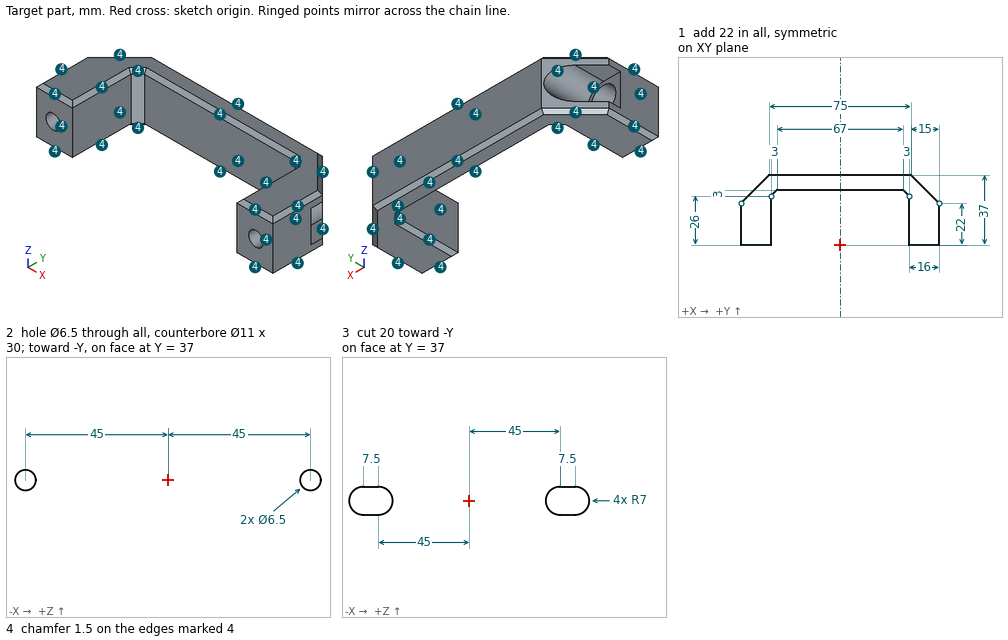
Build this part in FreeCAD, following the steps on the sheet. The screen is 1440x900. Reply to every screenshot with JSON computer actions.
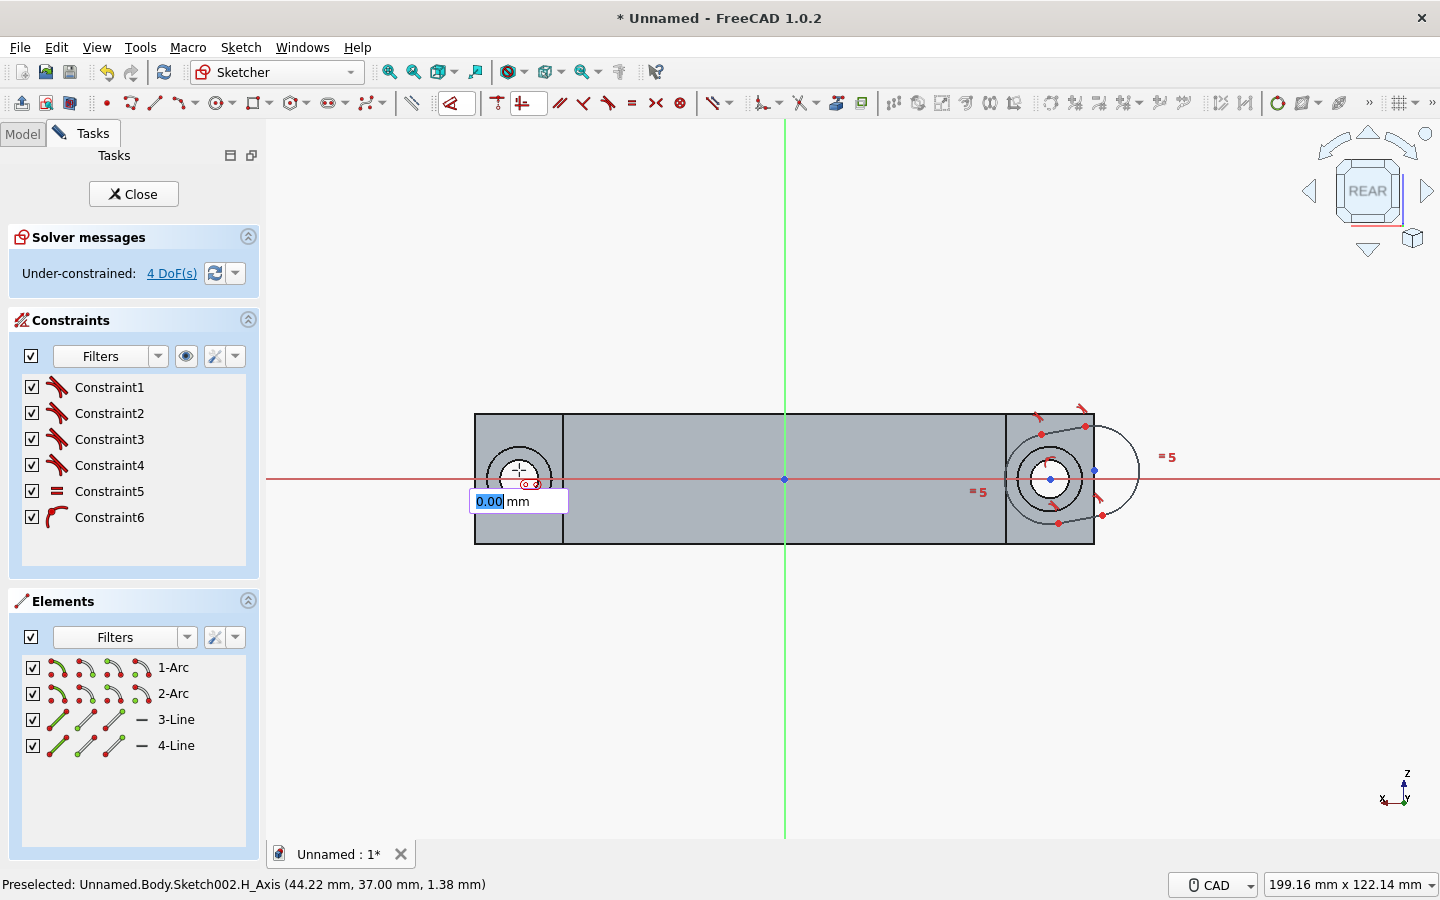
{"action": "left_click", "coordinate": [497, 520]}
{"action": "key", "text": "Escape"}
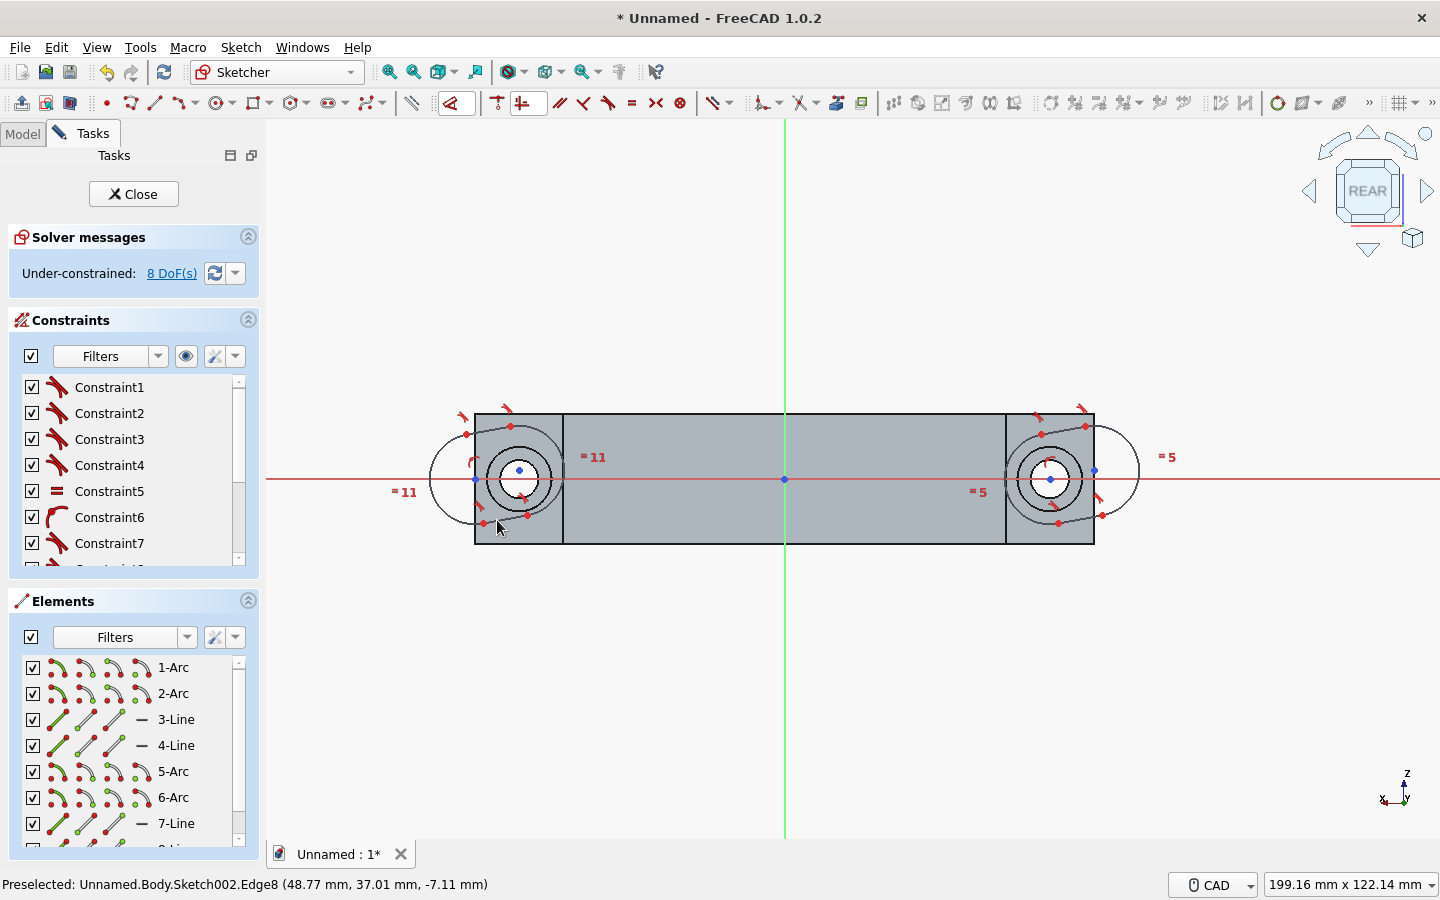
{"action": "left_click", "coordinate": [1055, 432]}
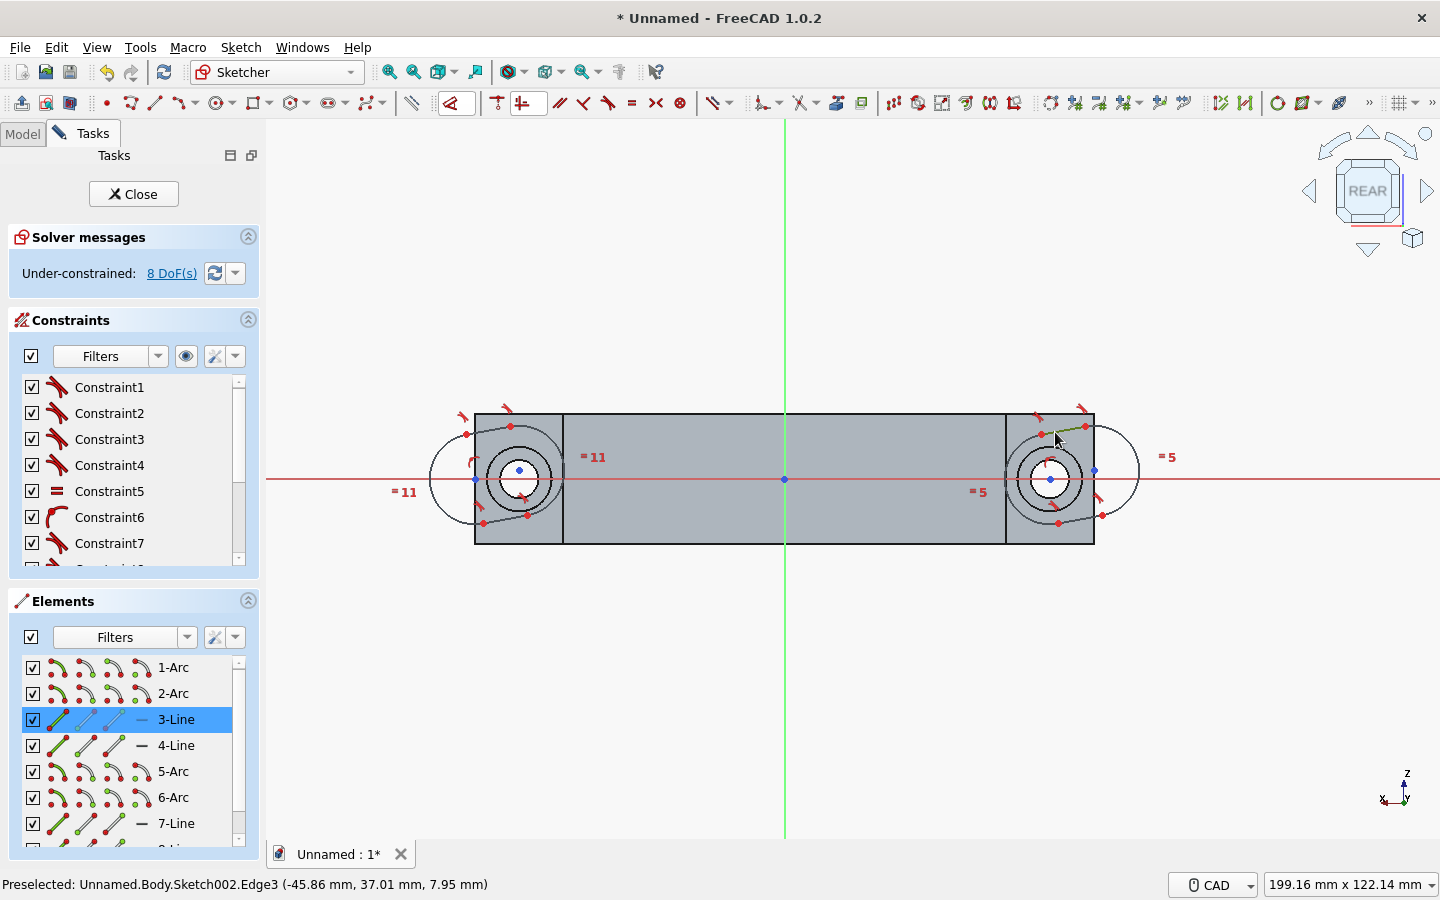
{"action": "key", "text": "h"}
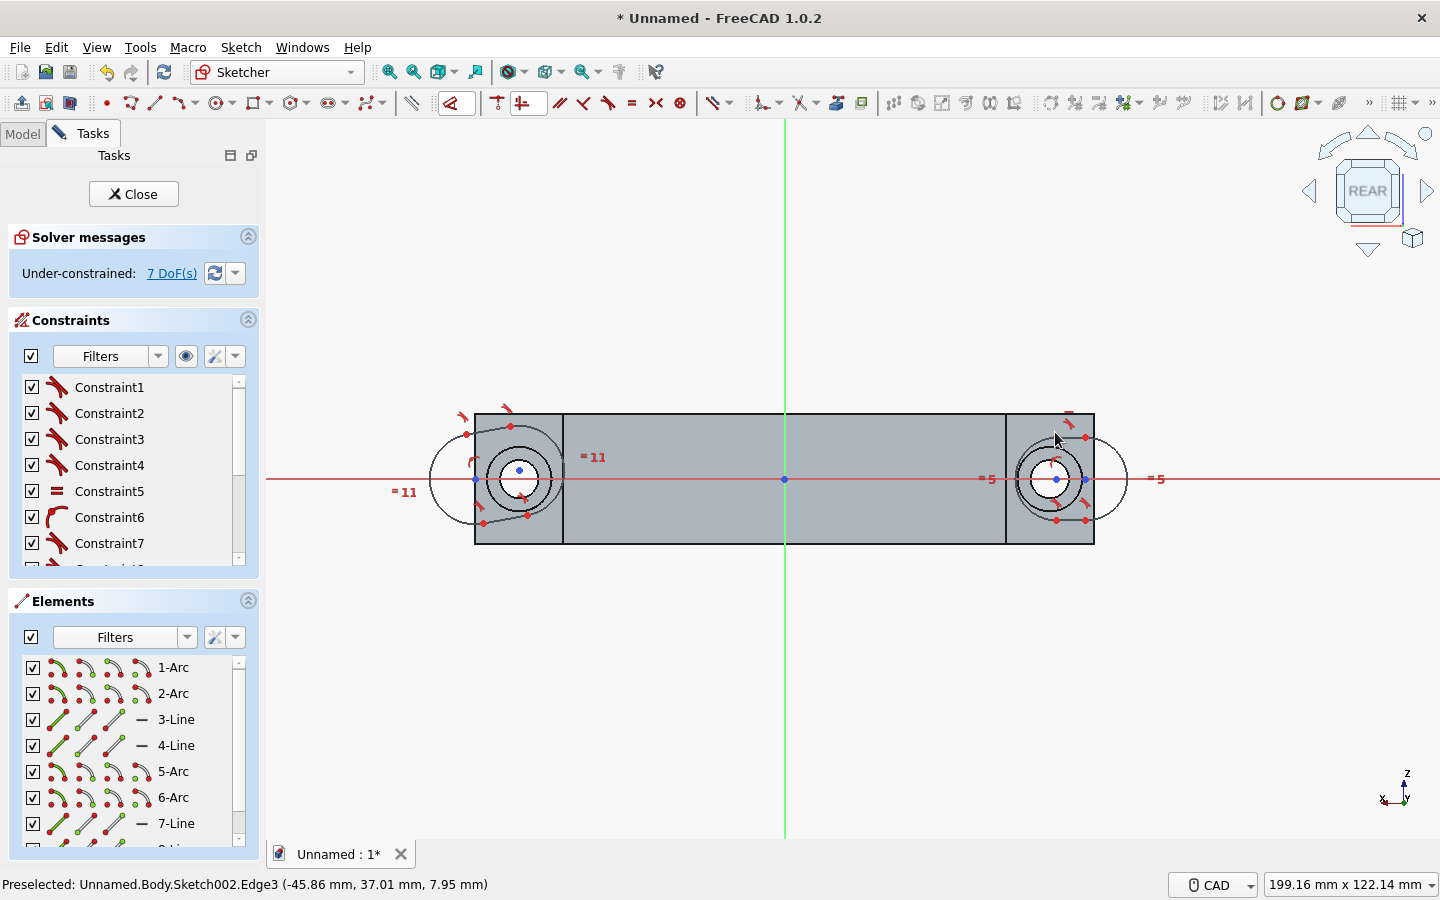
{"action": "left_click", "coordinate": [480, 432]}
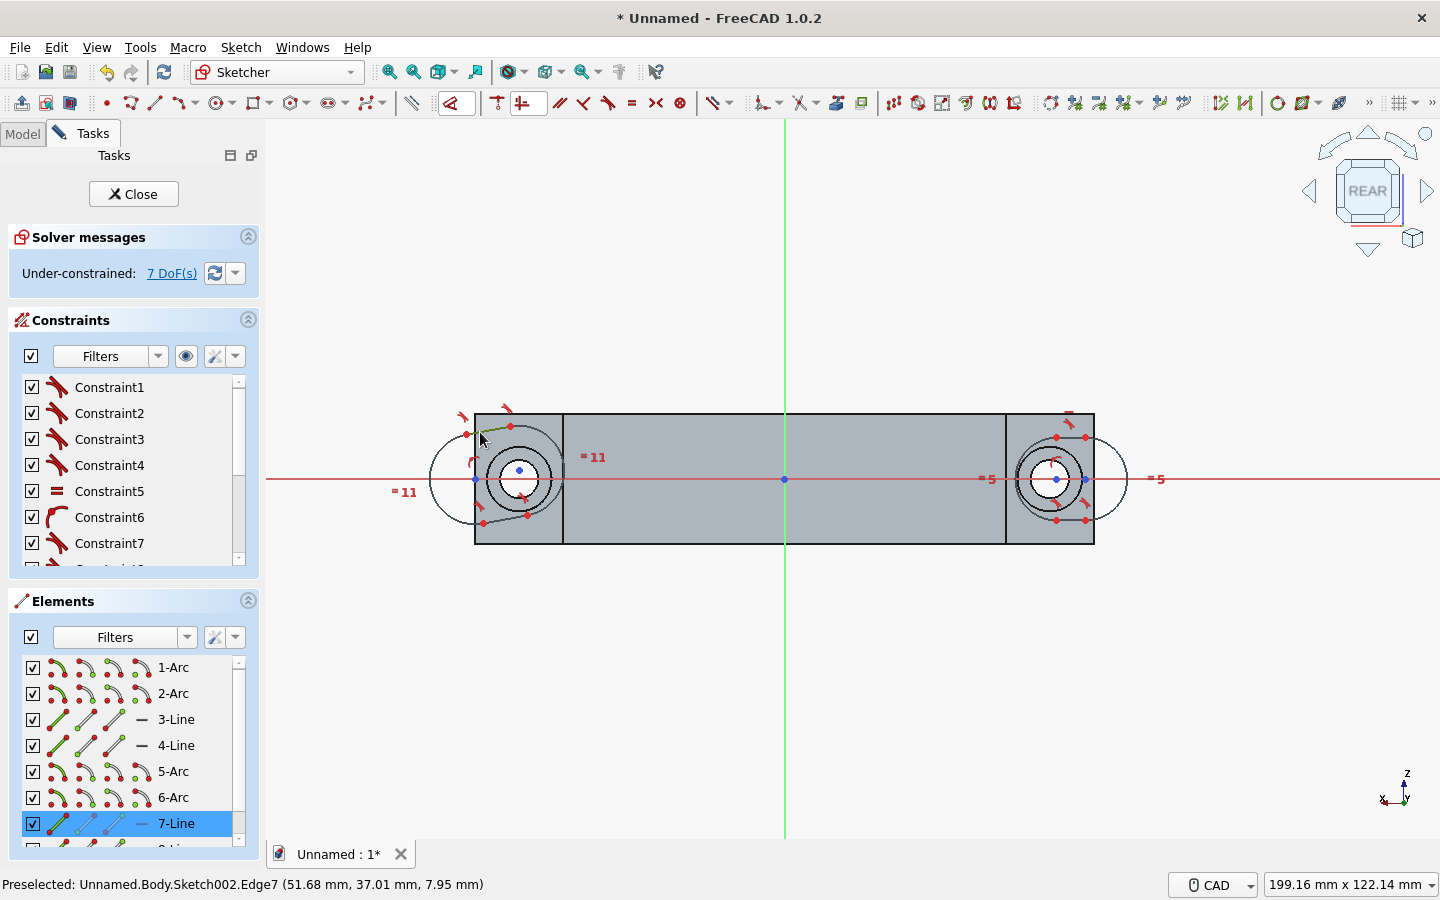
{"action": "left_click", "coordinate": [542, 104]}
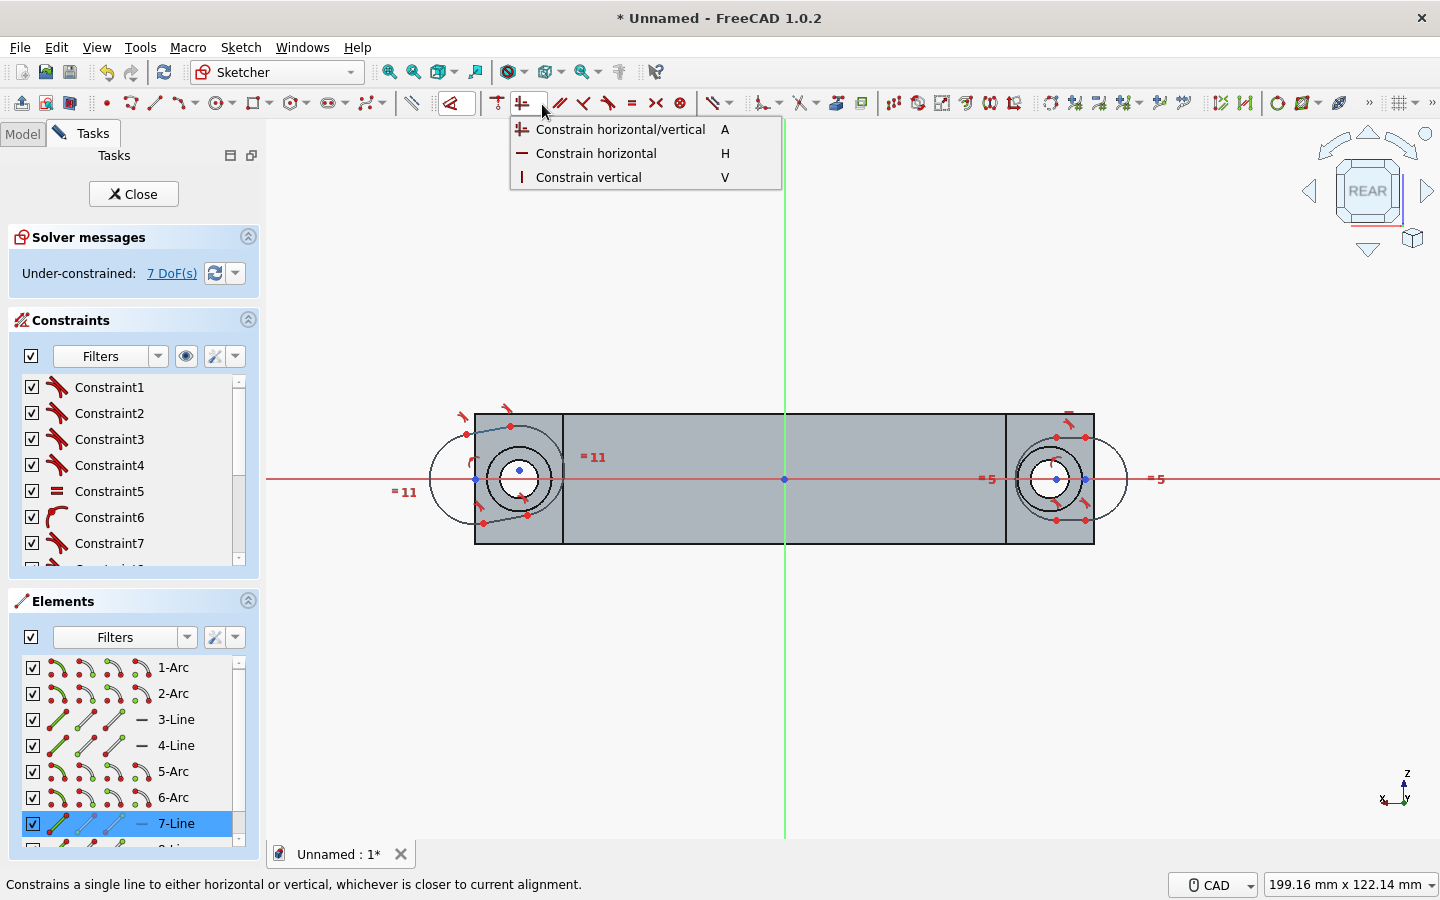
{"action": "left_click", "coordinate": [646, 153]}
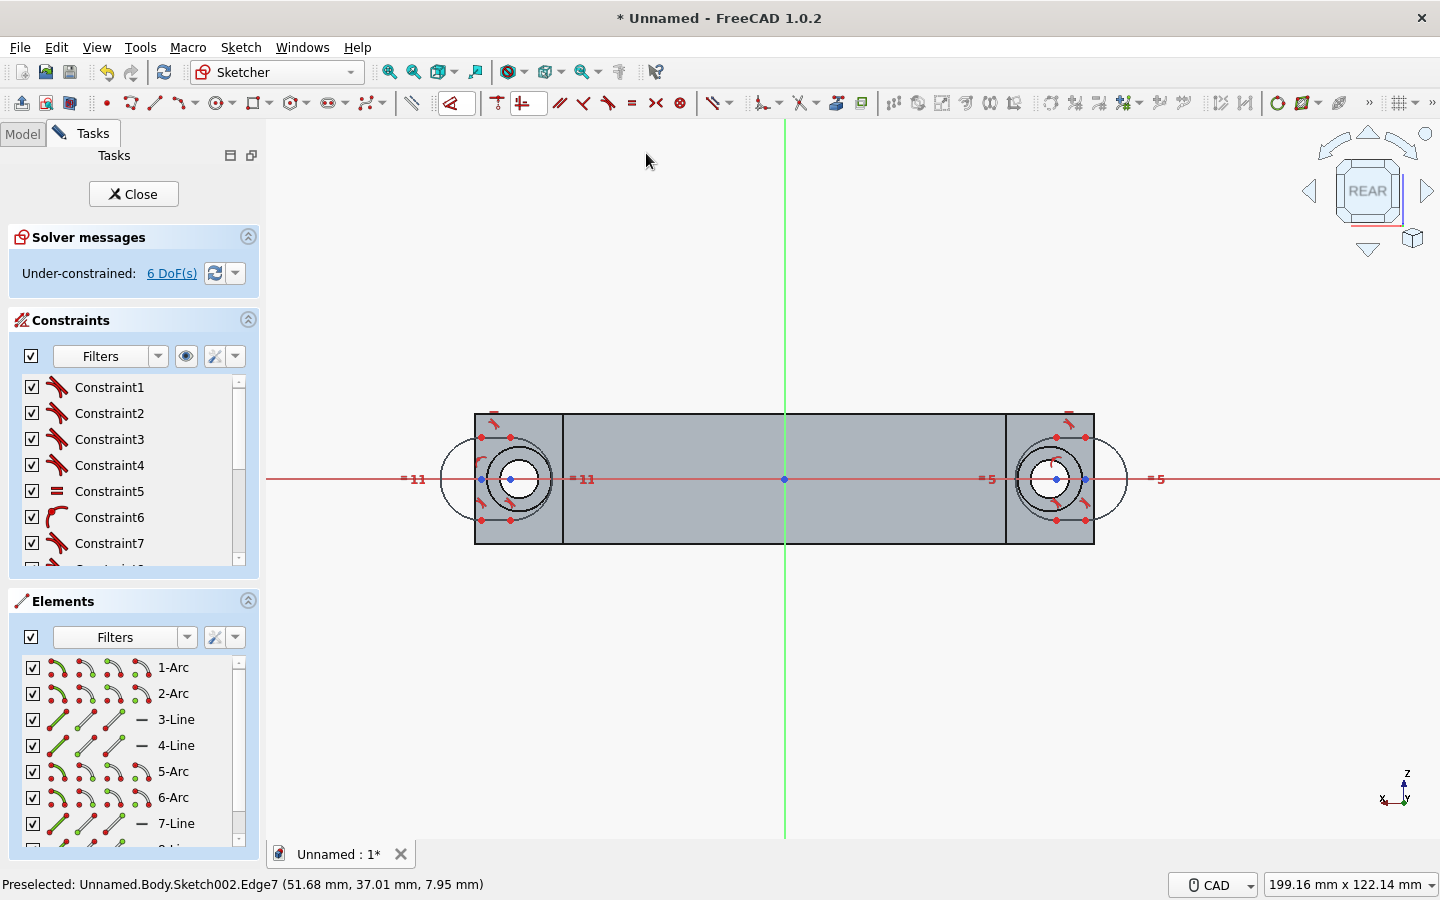
{"action": "left_click", "coordinate": [1023, 455]}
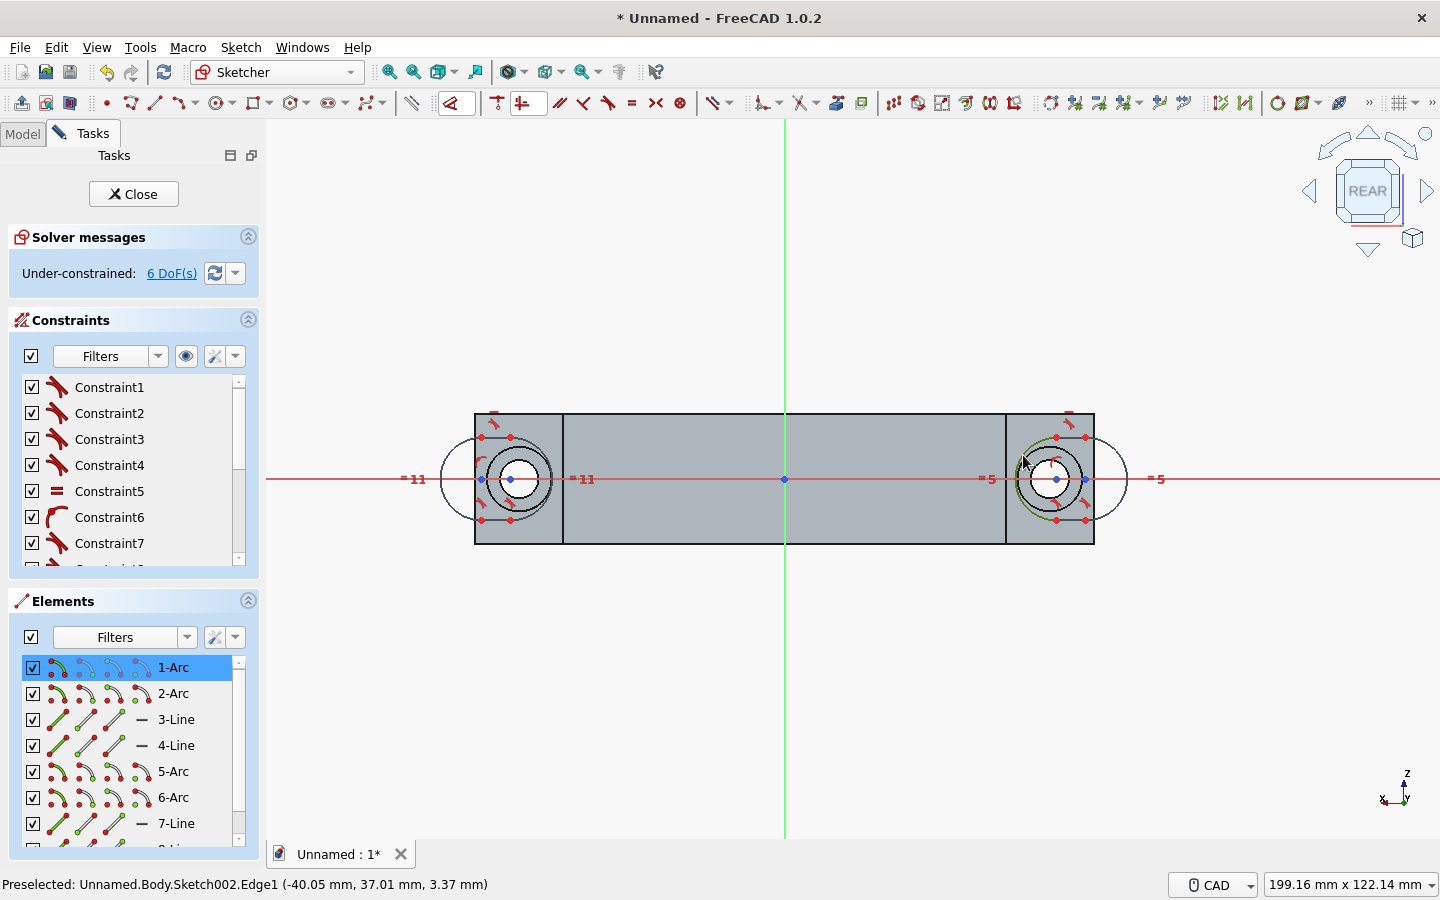
{"action": "left_click", "coordinate": [448, 455]}